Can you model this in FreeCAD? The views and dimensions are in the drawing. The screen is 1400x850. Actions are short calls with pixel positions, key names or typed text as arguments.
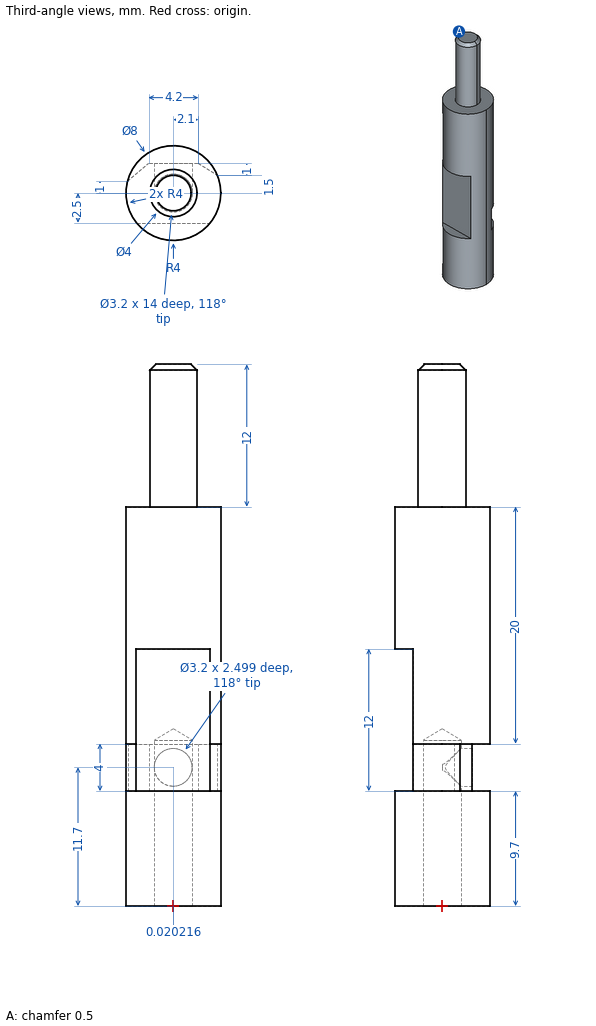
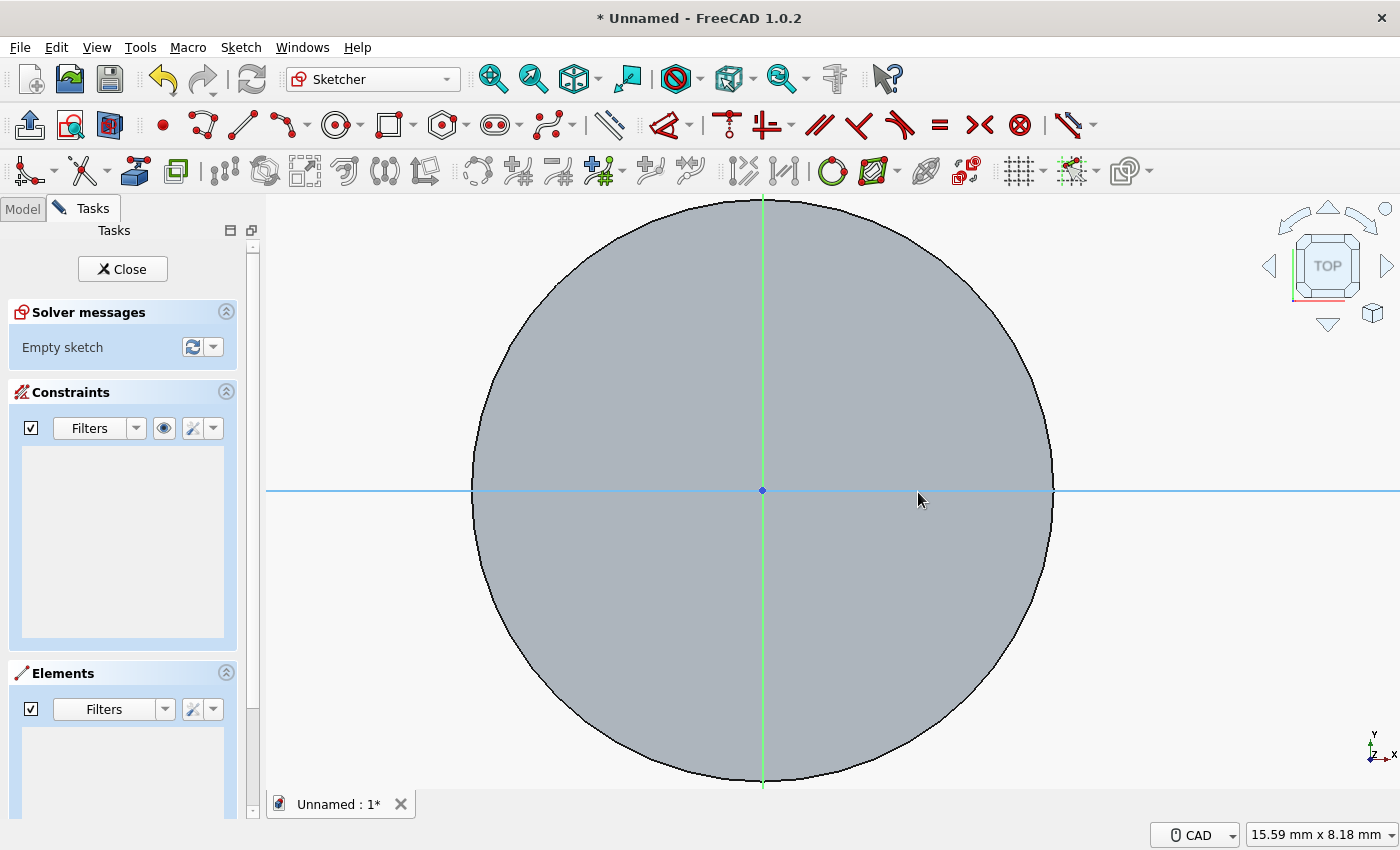
click(244, 126)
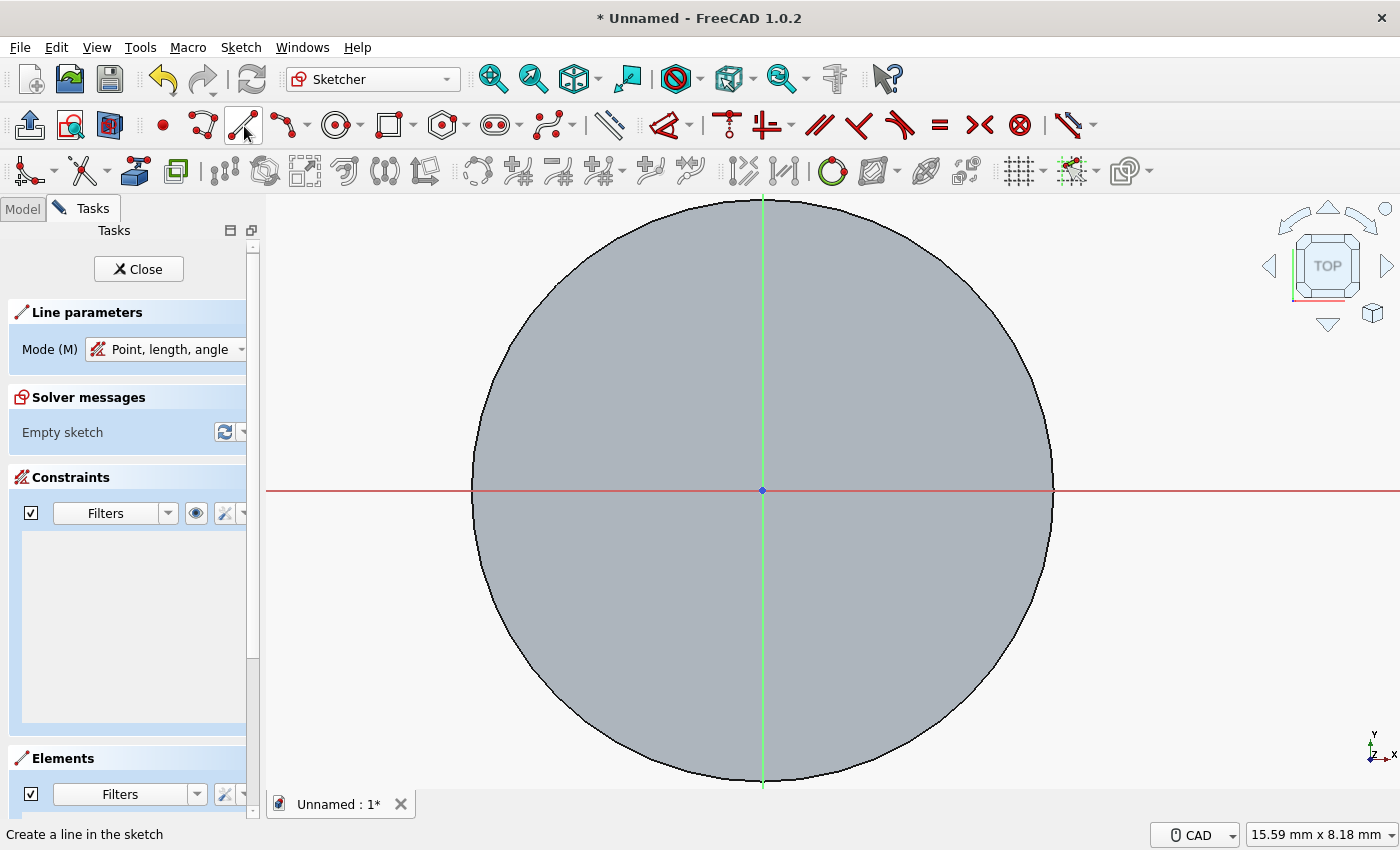
click(535, 673)
click(990, 673)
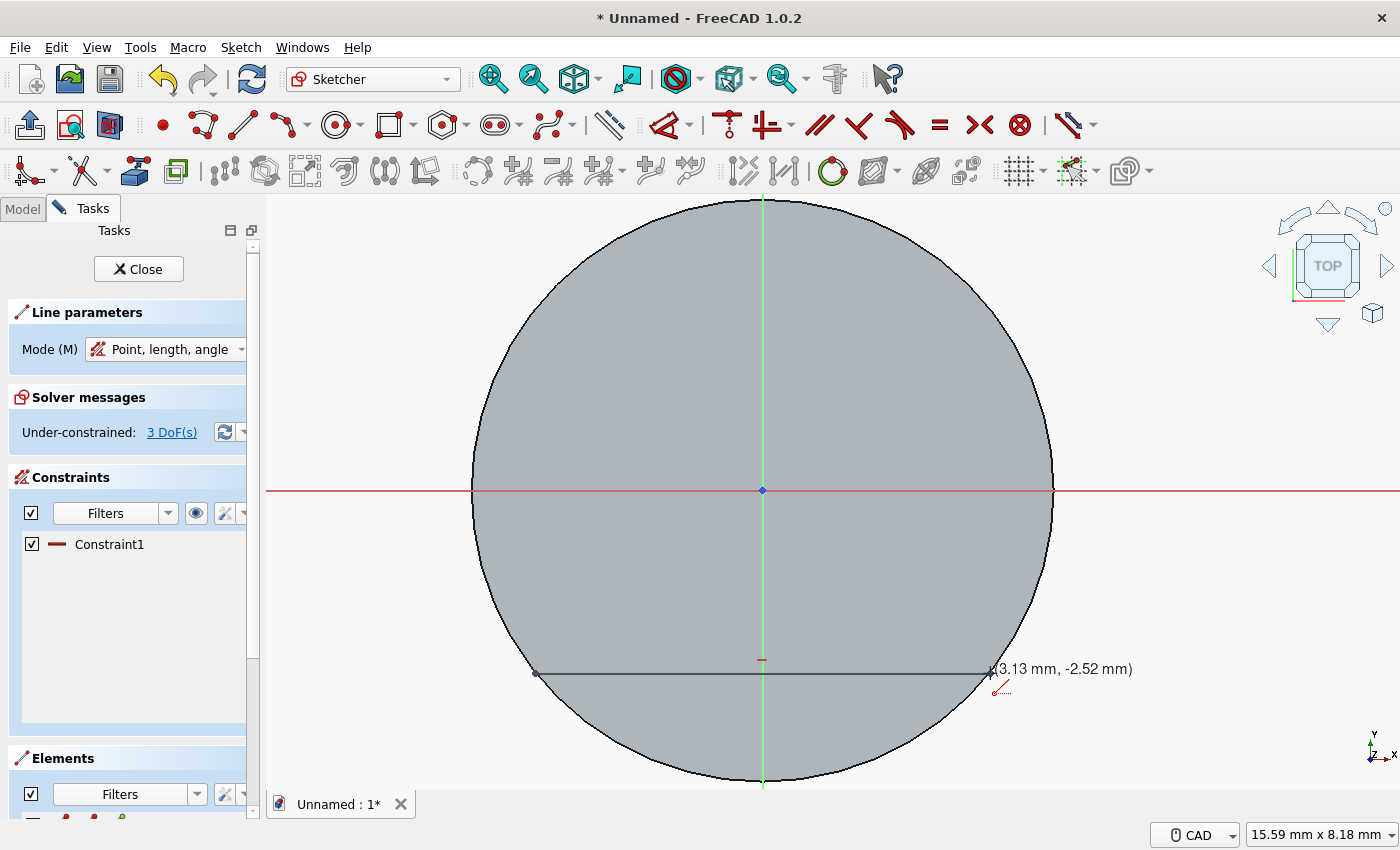
key(g)
key(m)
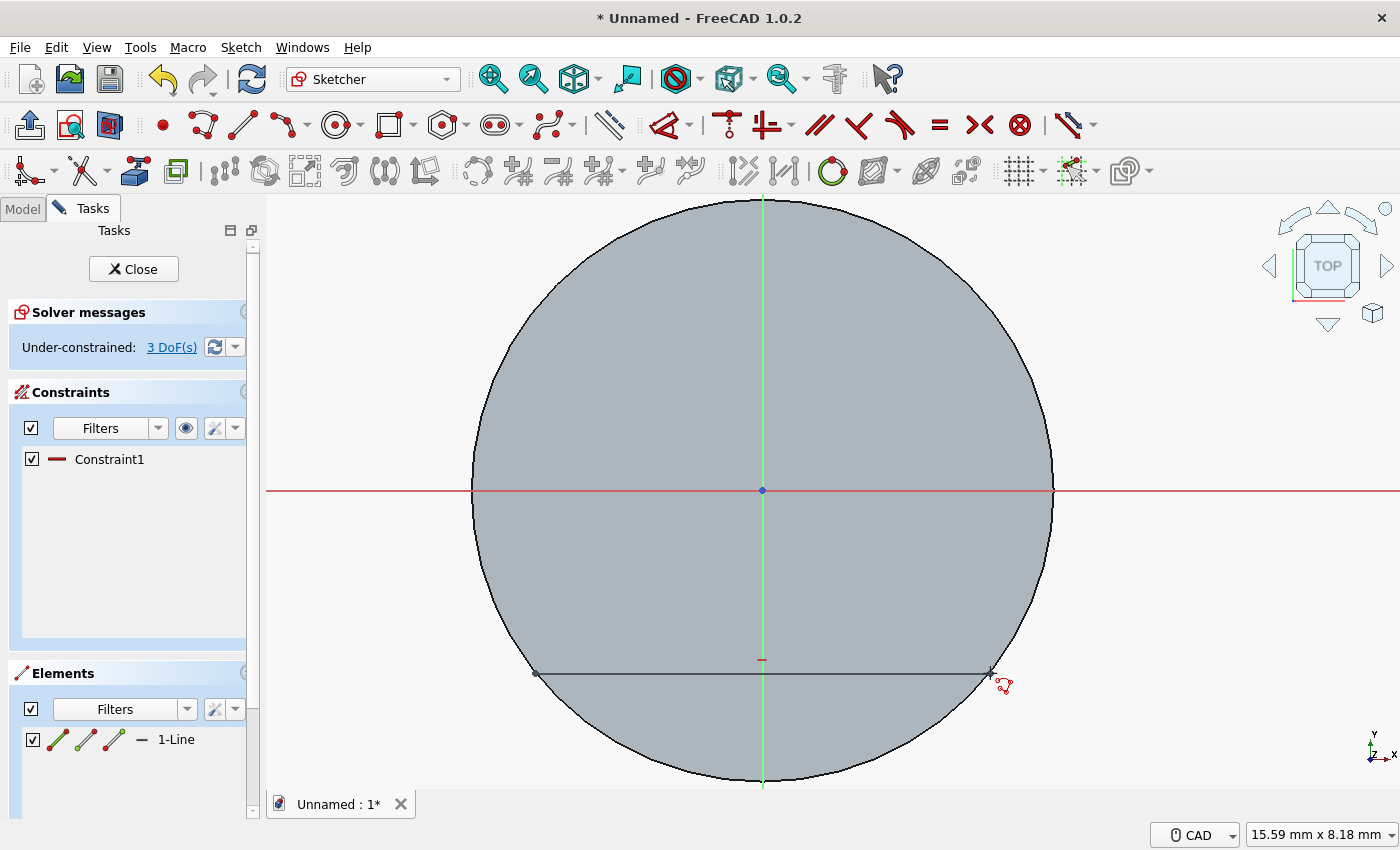
click(1032, 382)
click(915, 309)
click(610, 309)
click(481, 418)
right_click(481, 418)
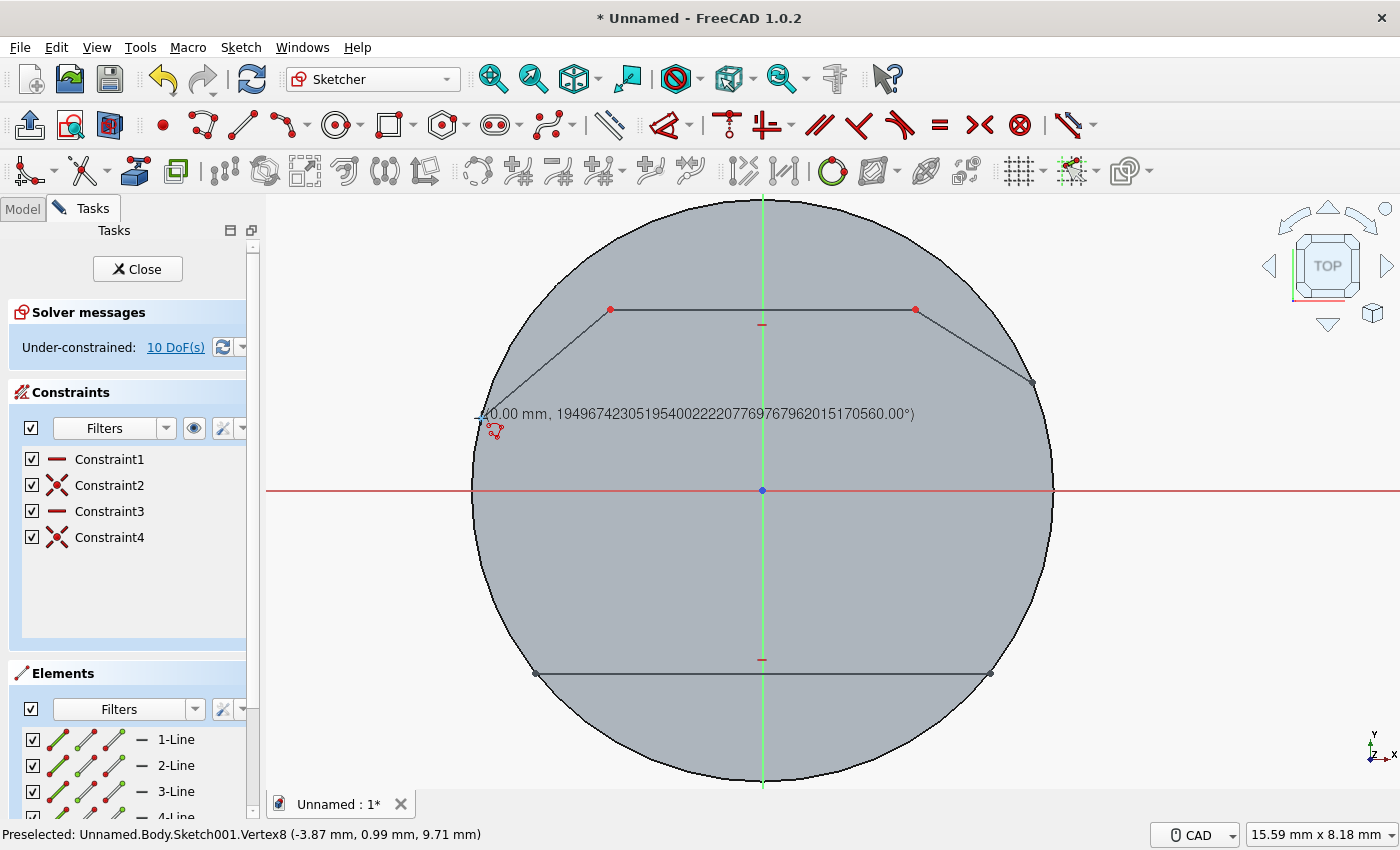
key(g)
key(3)
key(a)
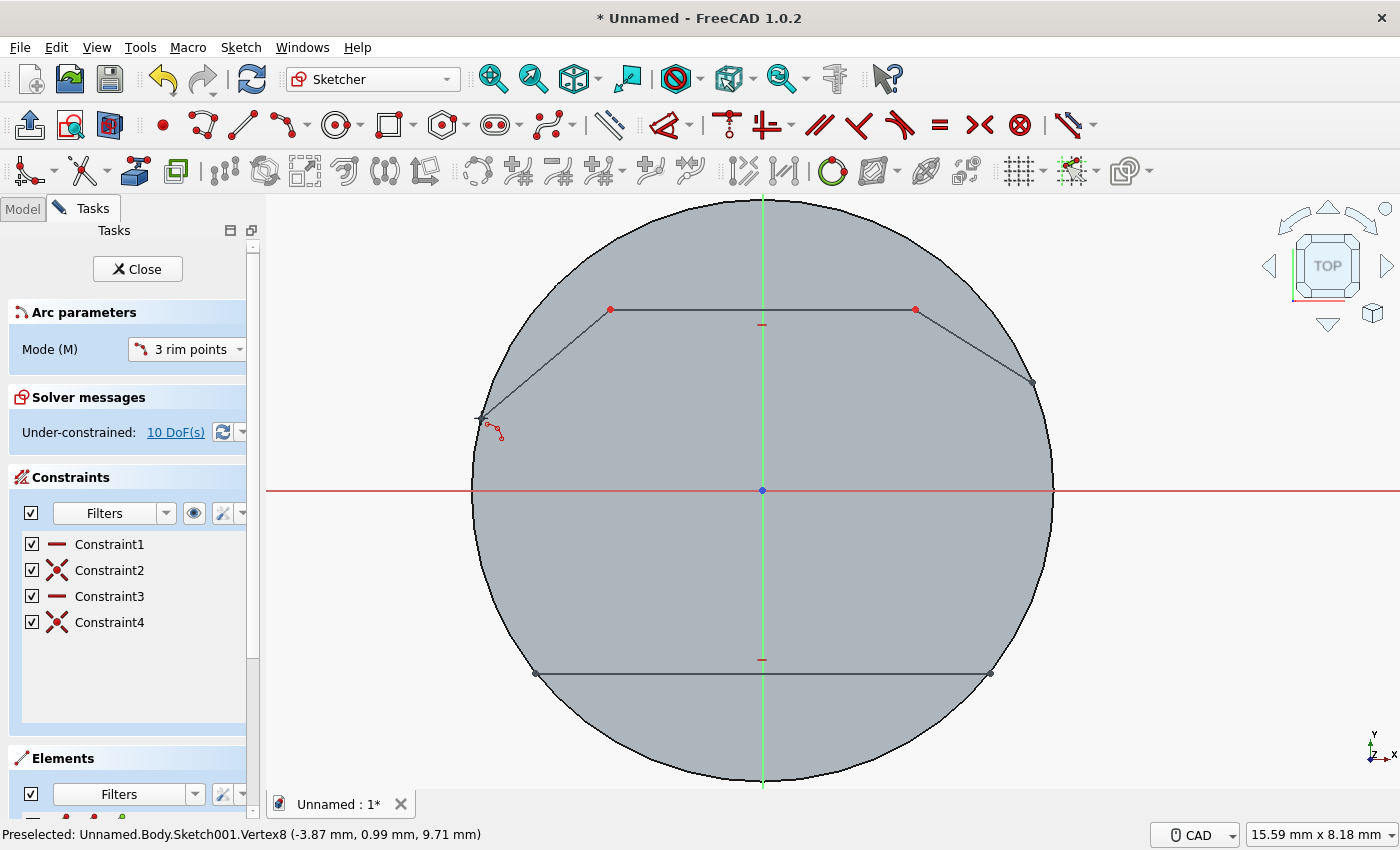
click(990, 674)
click(1032, 383)
click(1051, 533)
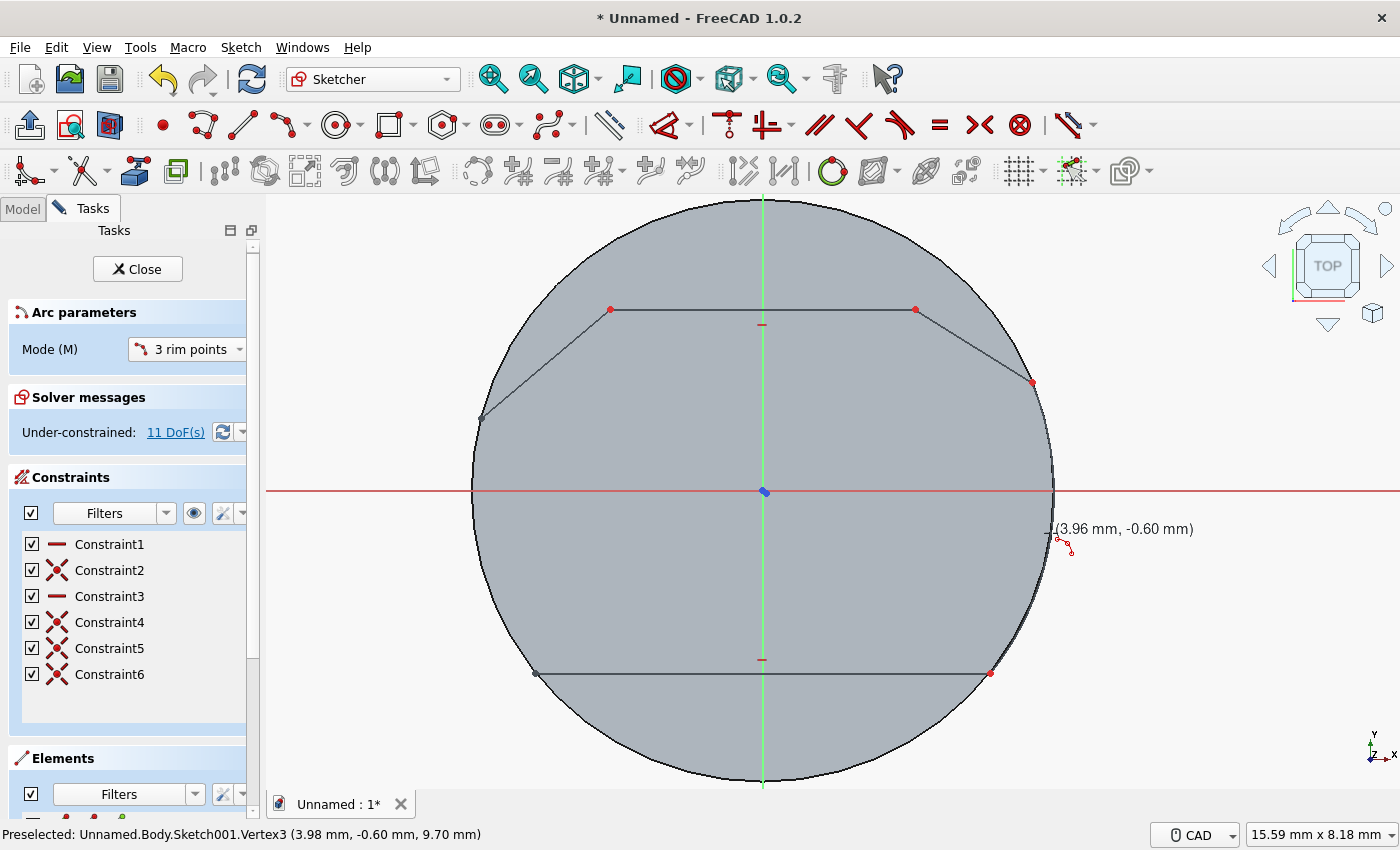
click(481, 419)
click(535, 674)
click(478, 552)
key(Escape)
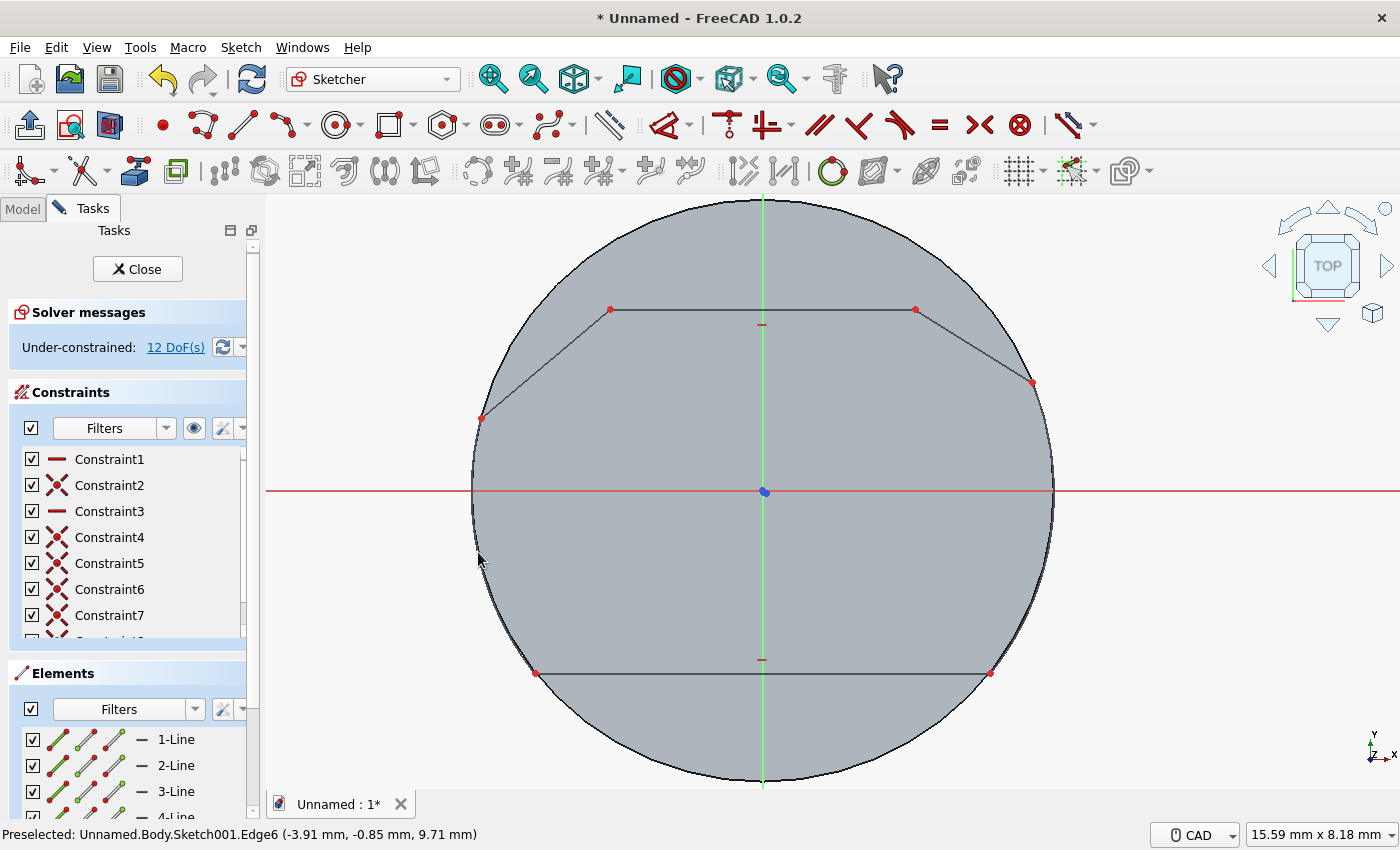
click(1036, 594)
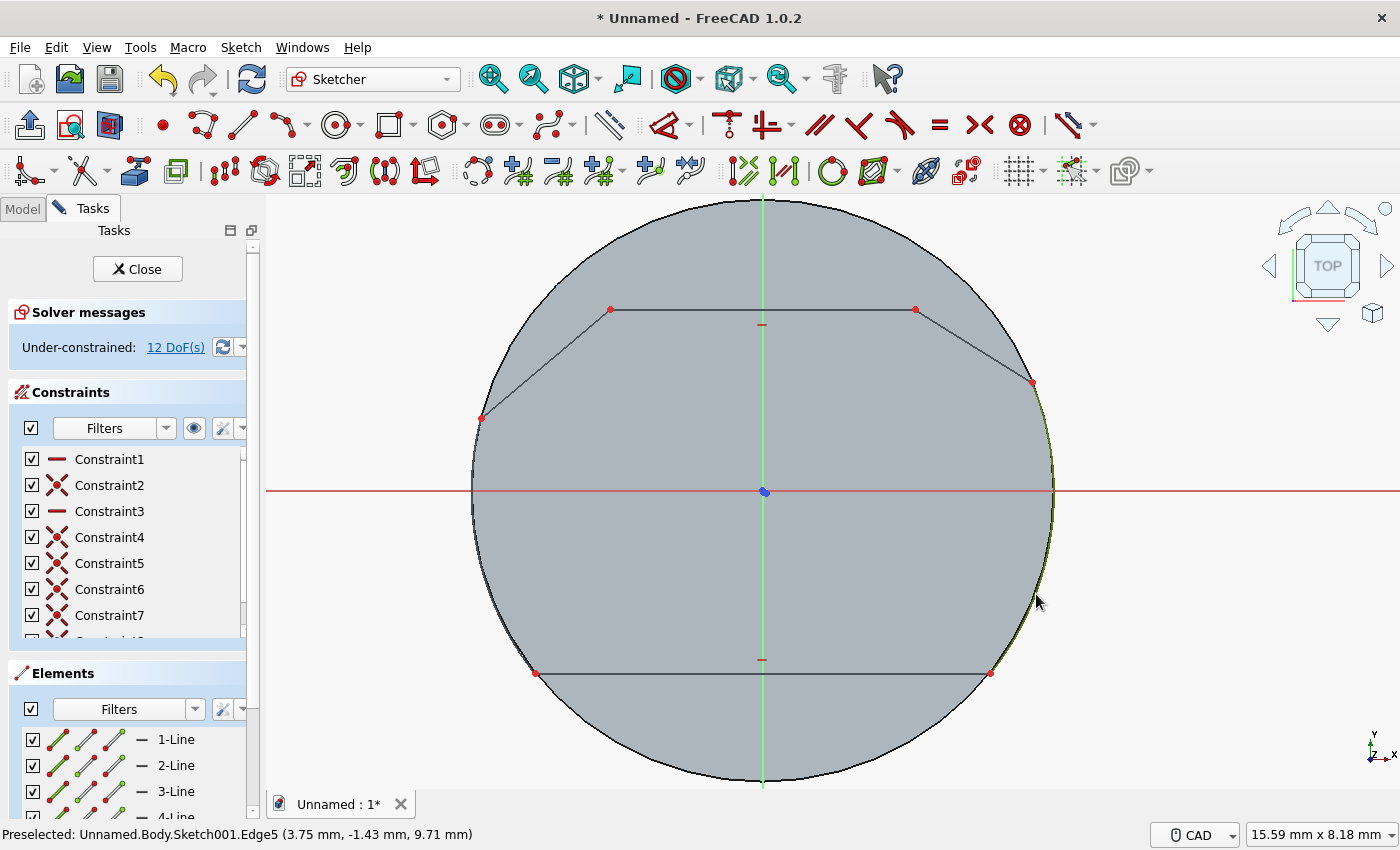
click(494, 604)